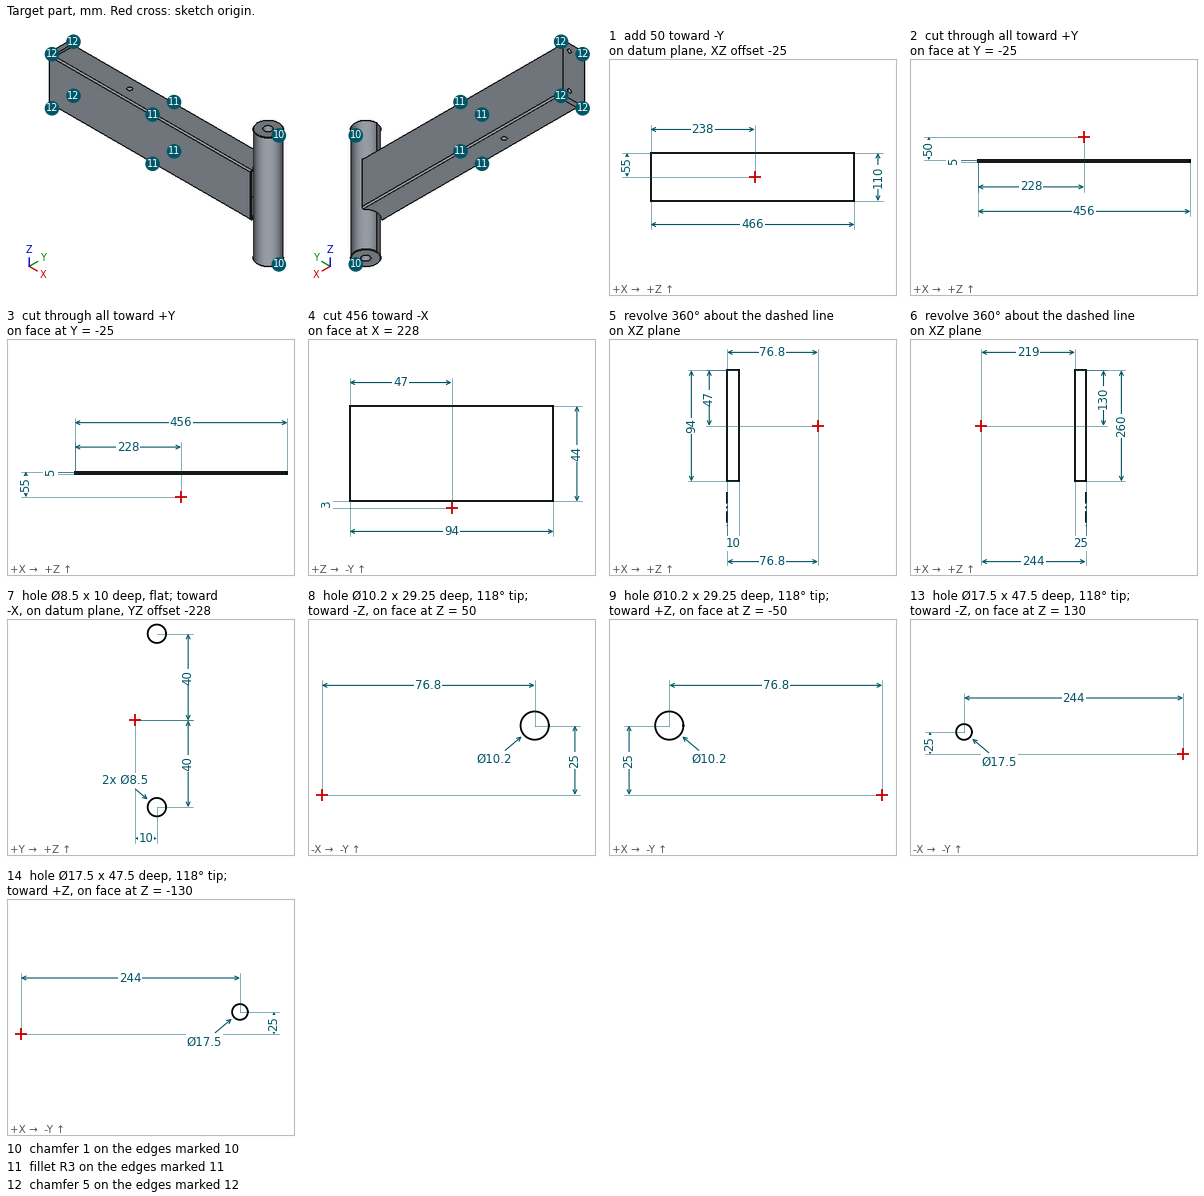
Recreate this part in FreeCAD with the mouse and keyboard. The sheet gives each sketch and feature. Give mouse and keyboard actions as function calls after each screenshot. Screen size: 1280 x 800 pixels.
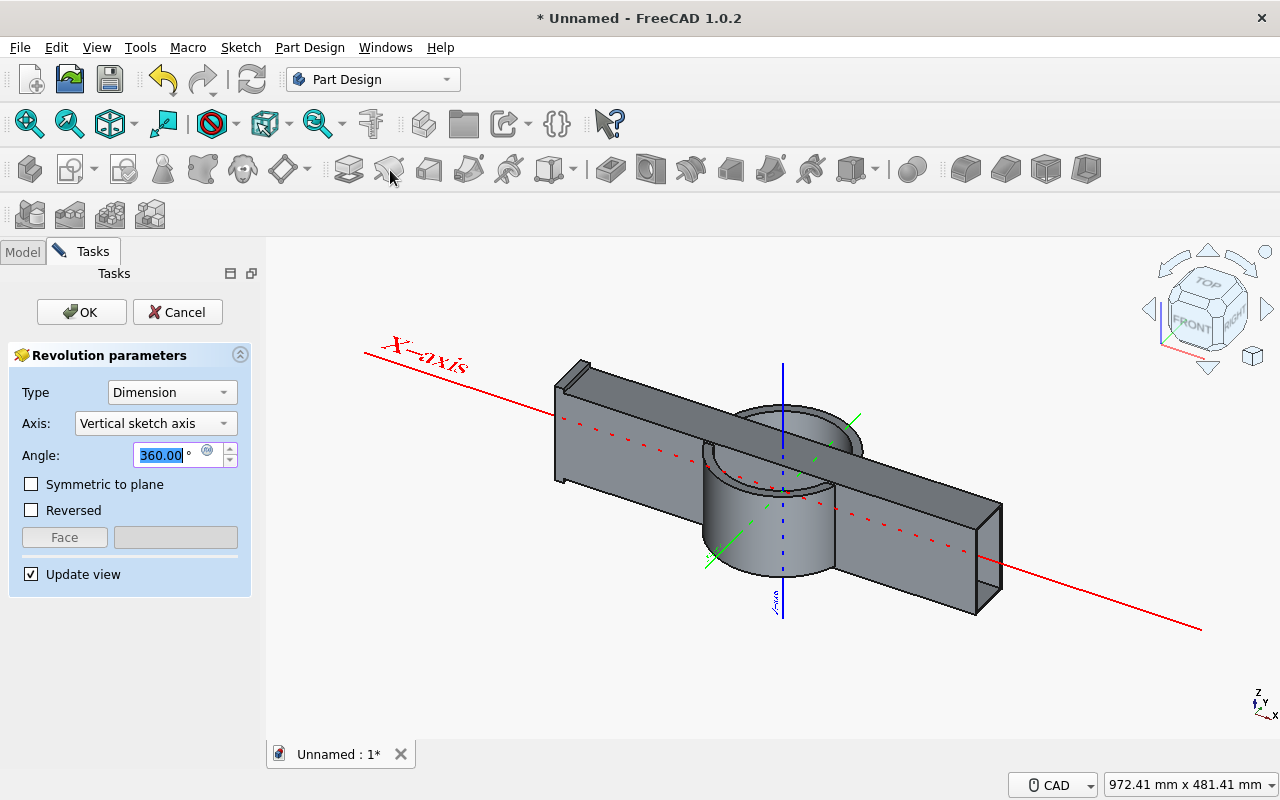
click(156, 424)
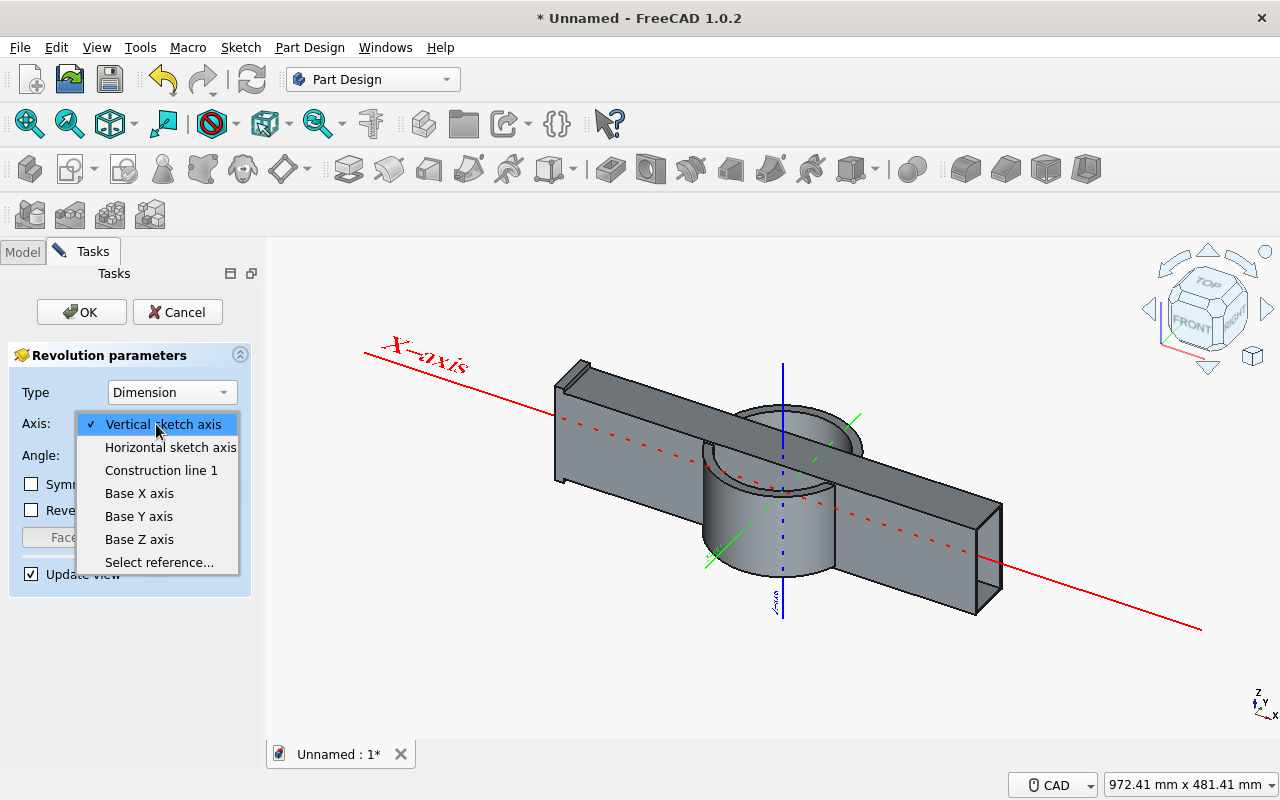
click(156, 470)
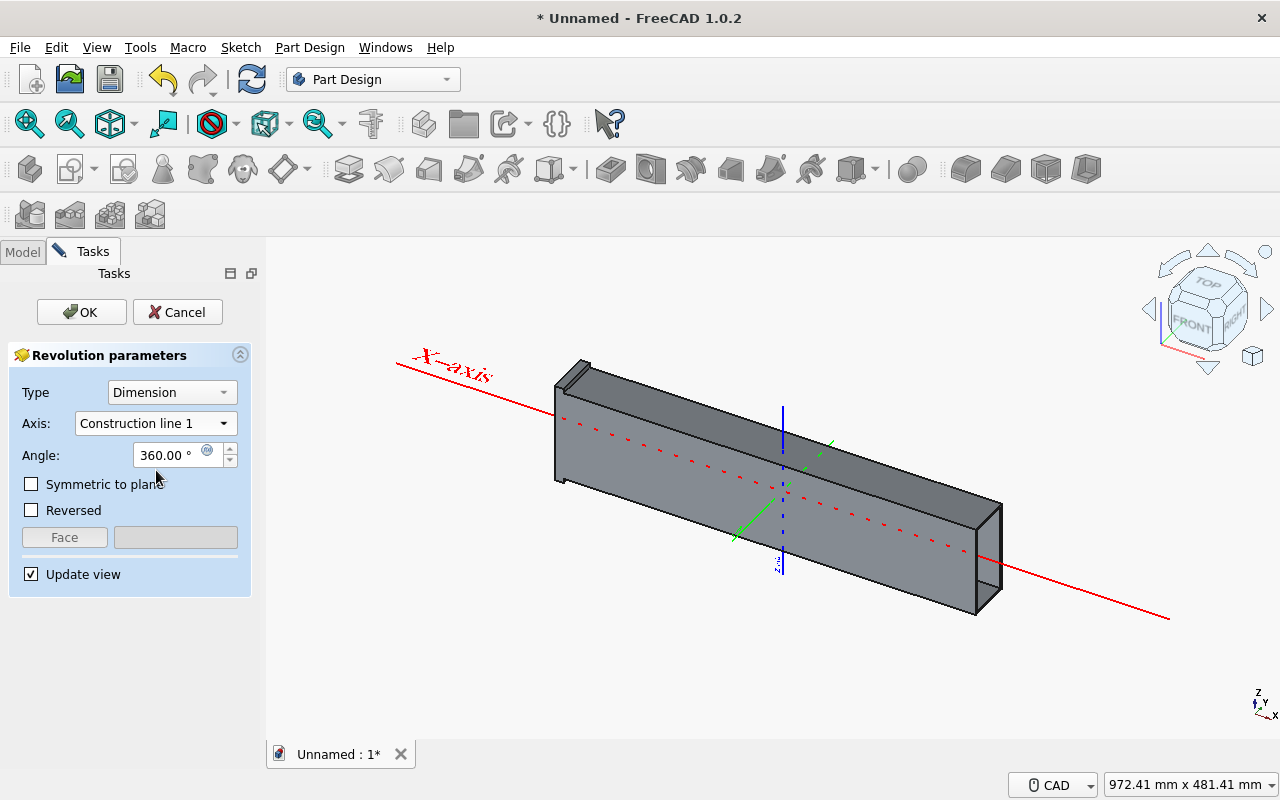
click(82, 312)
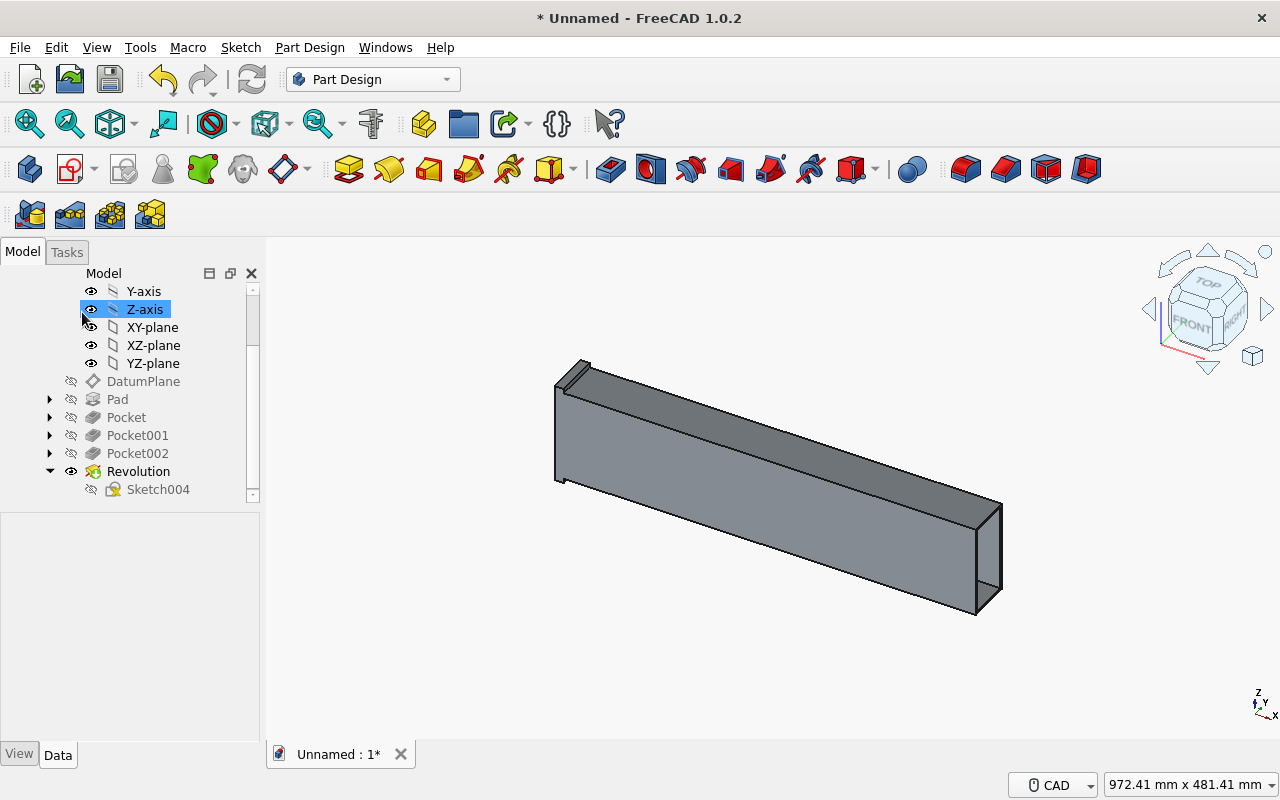
click(70, 170)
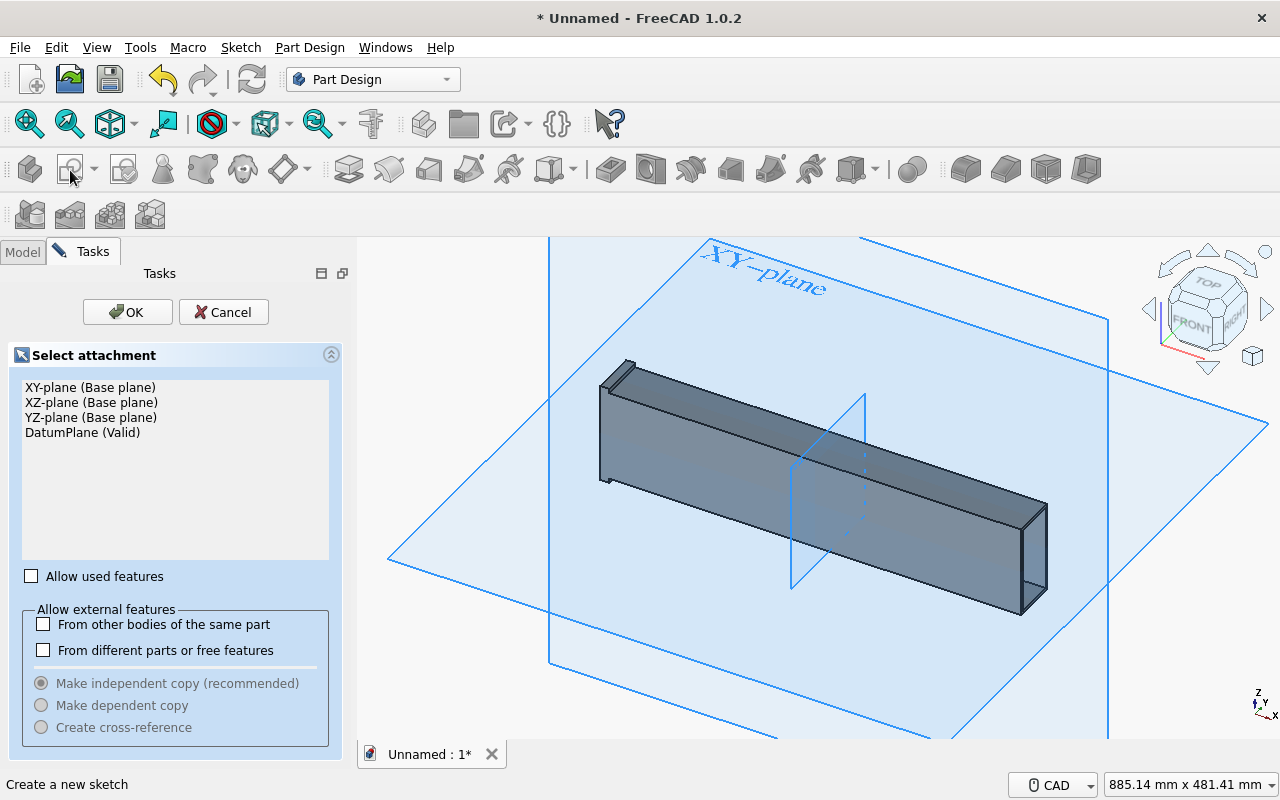
click(82, 402)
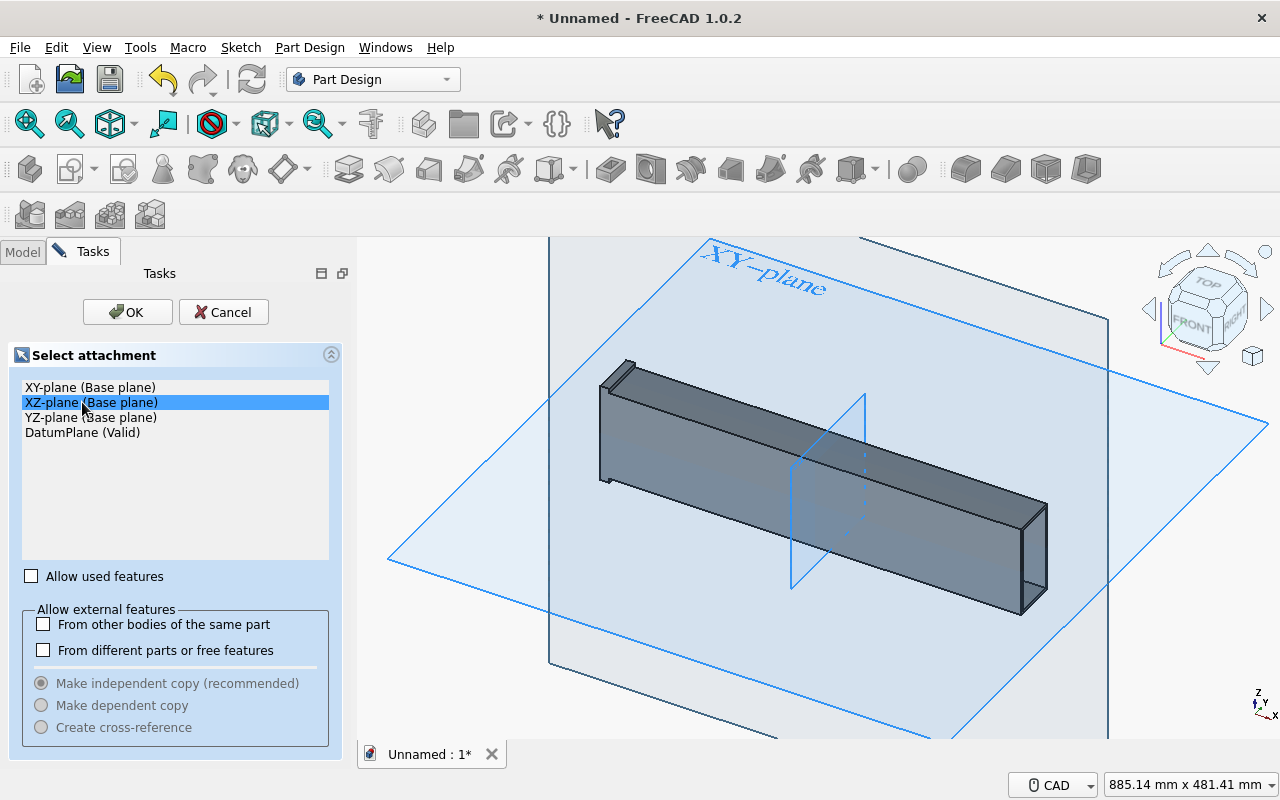
click(128, 312)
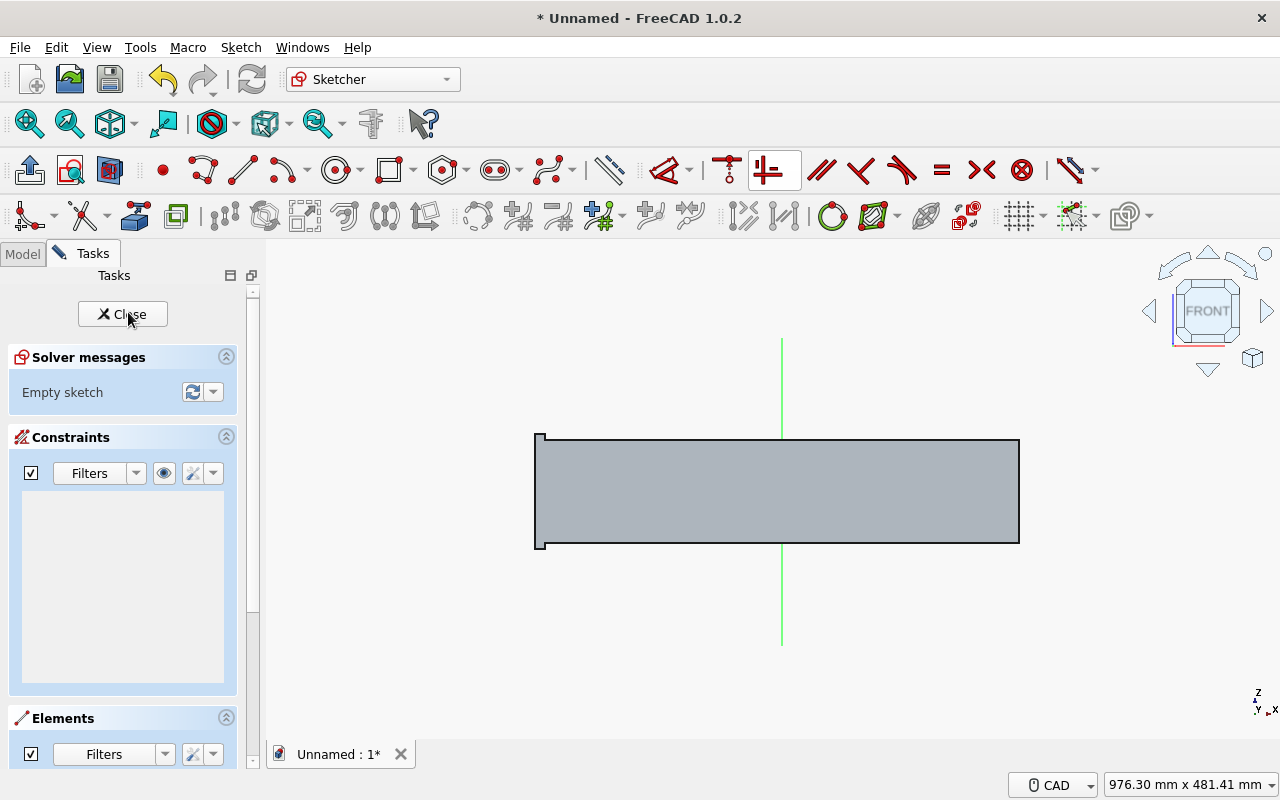
click(110, 170)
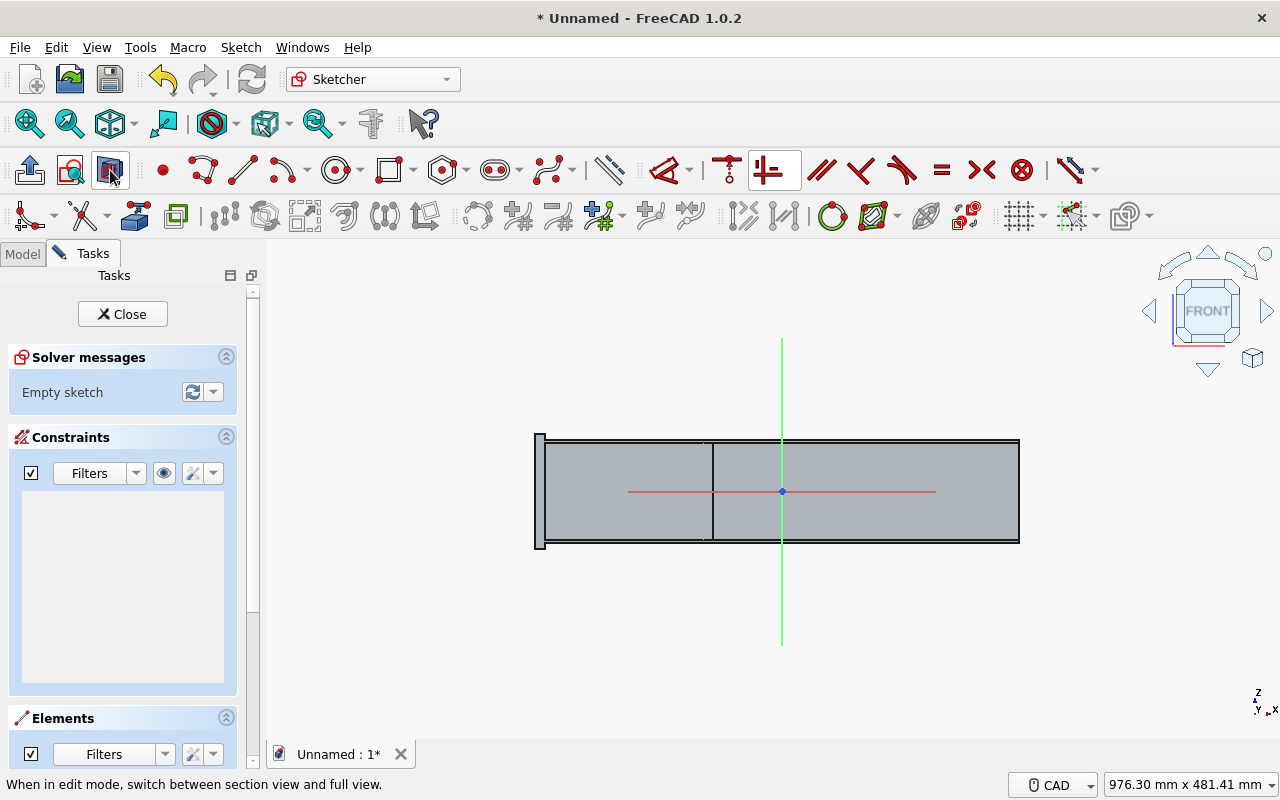
scroll(294, 267, down, 1)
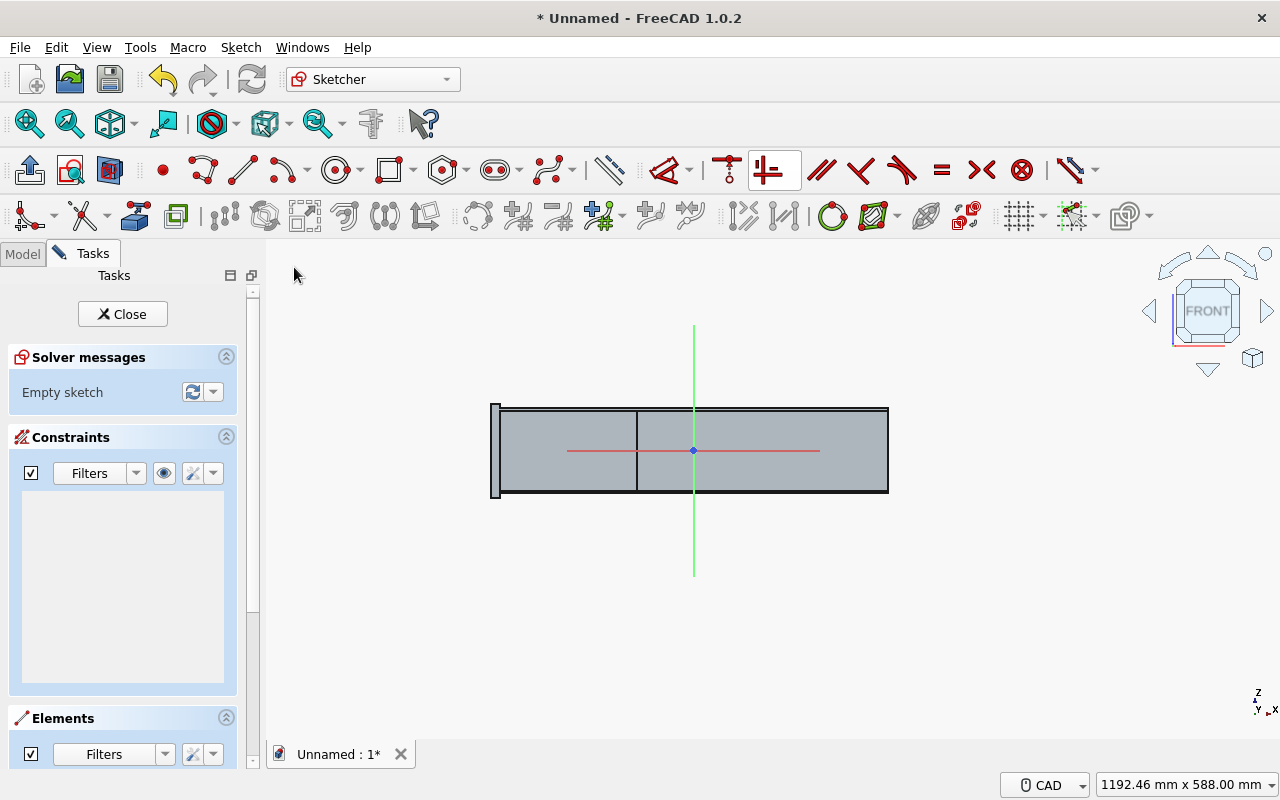
click(390, 170)